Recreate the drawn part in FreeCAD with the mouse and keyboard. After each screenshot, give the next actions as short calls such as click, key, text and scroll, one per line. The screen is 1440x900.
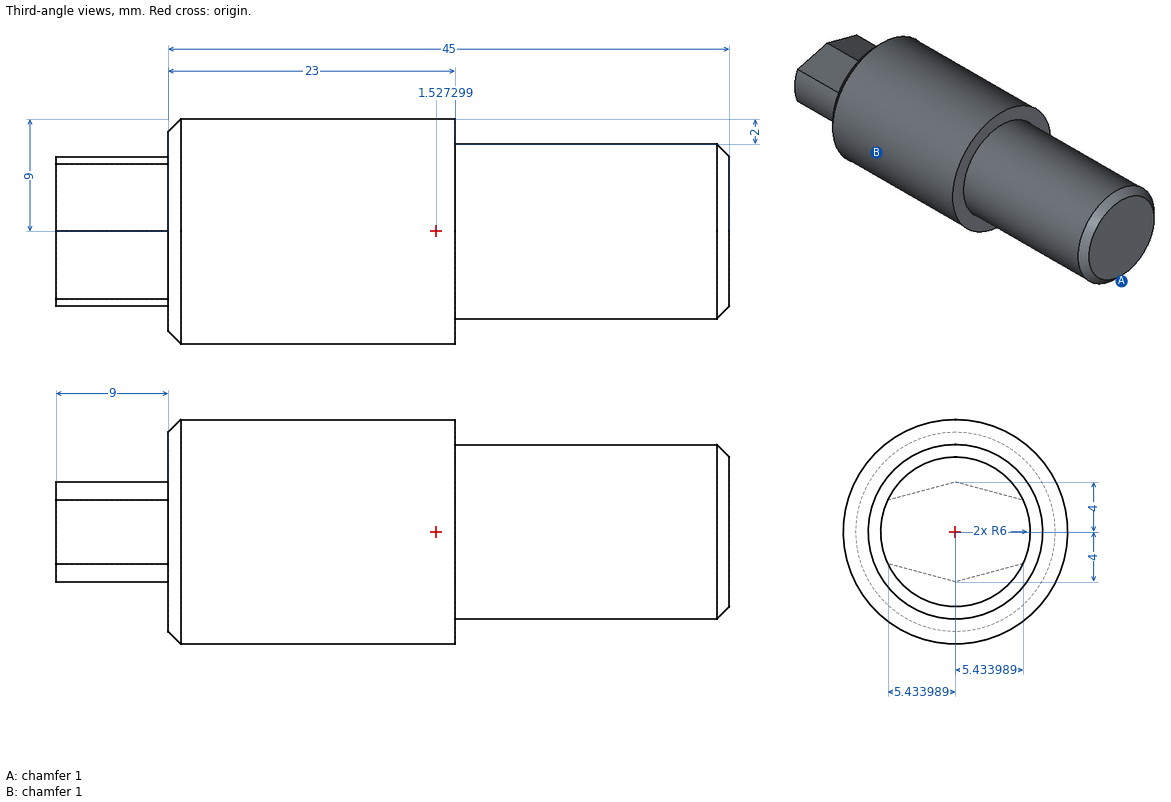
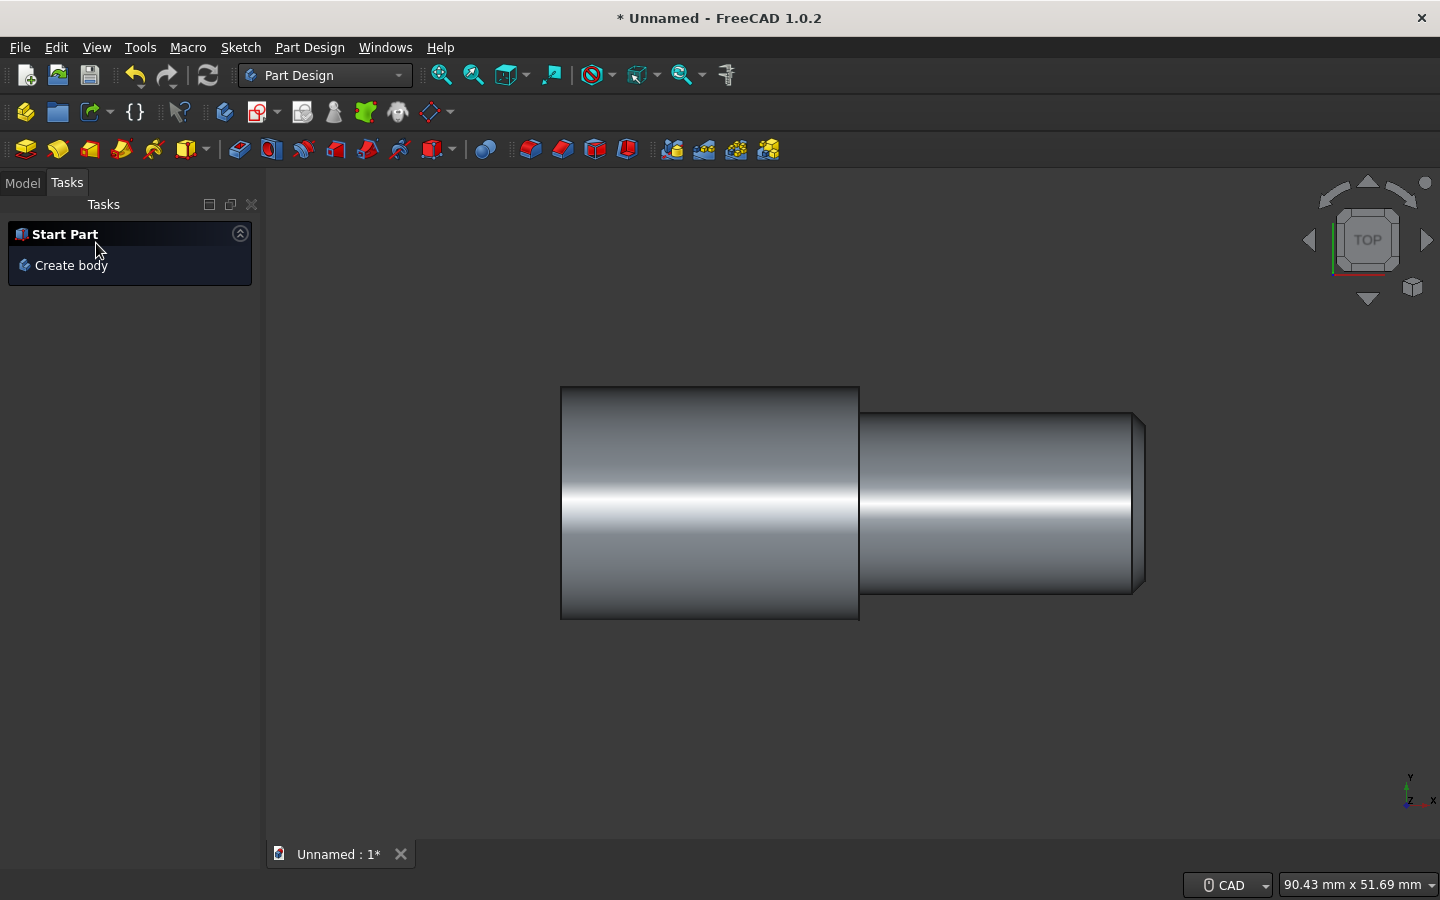
click(561, 597)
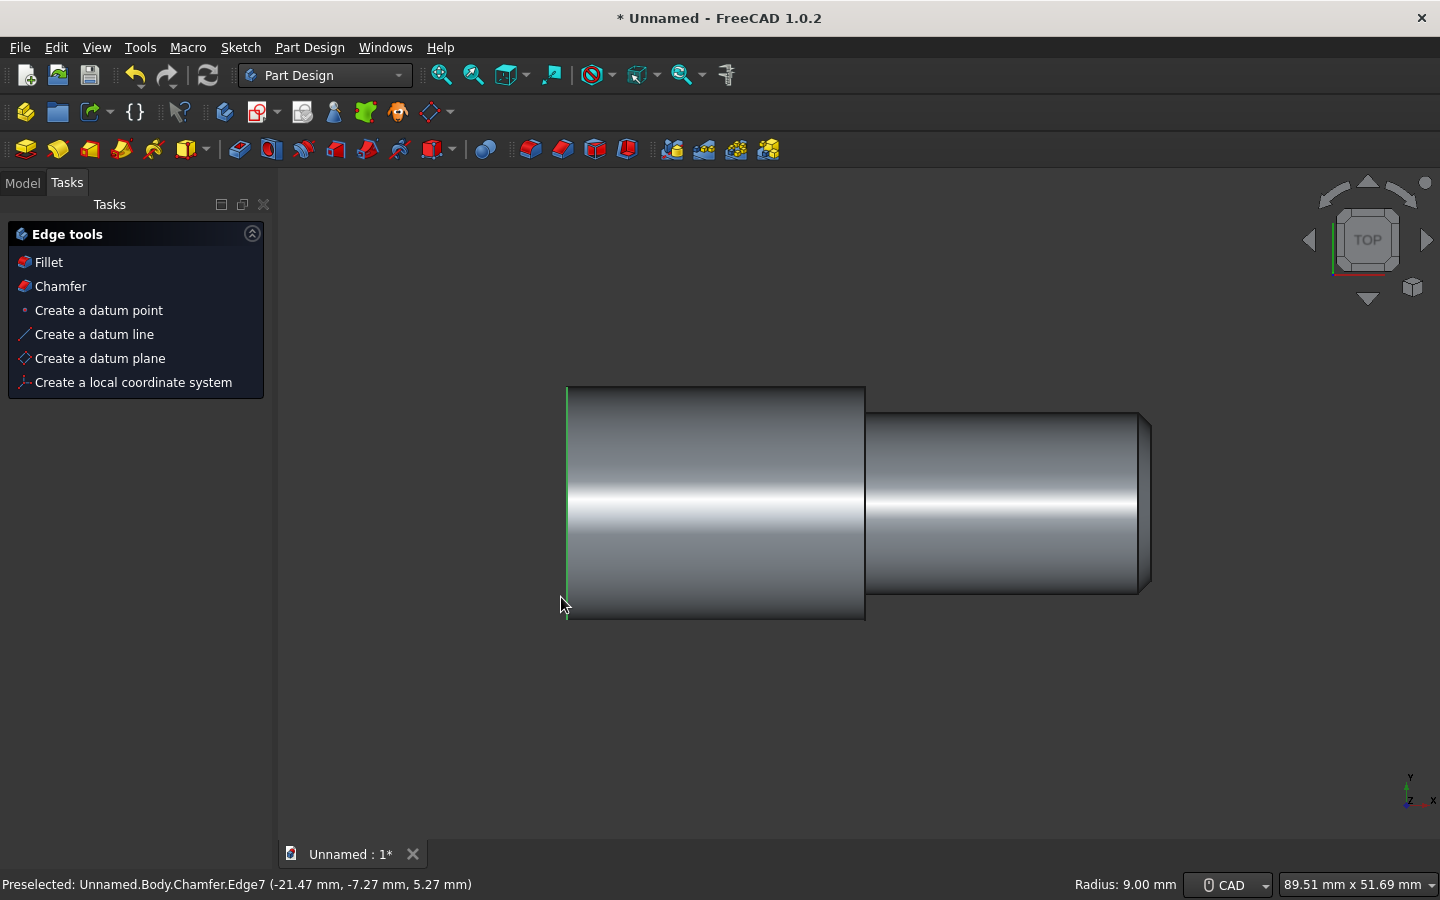
click(564, 150)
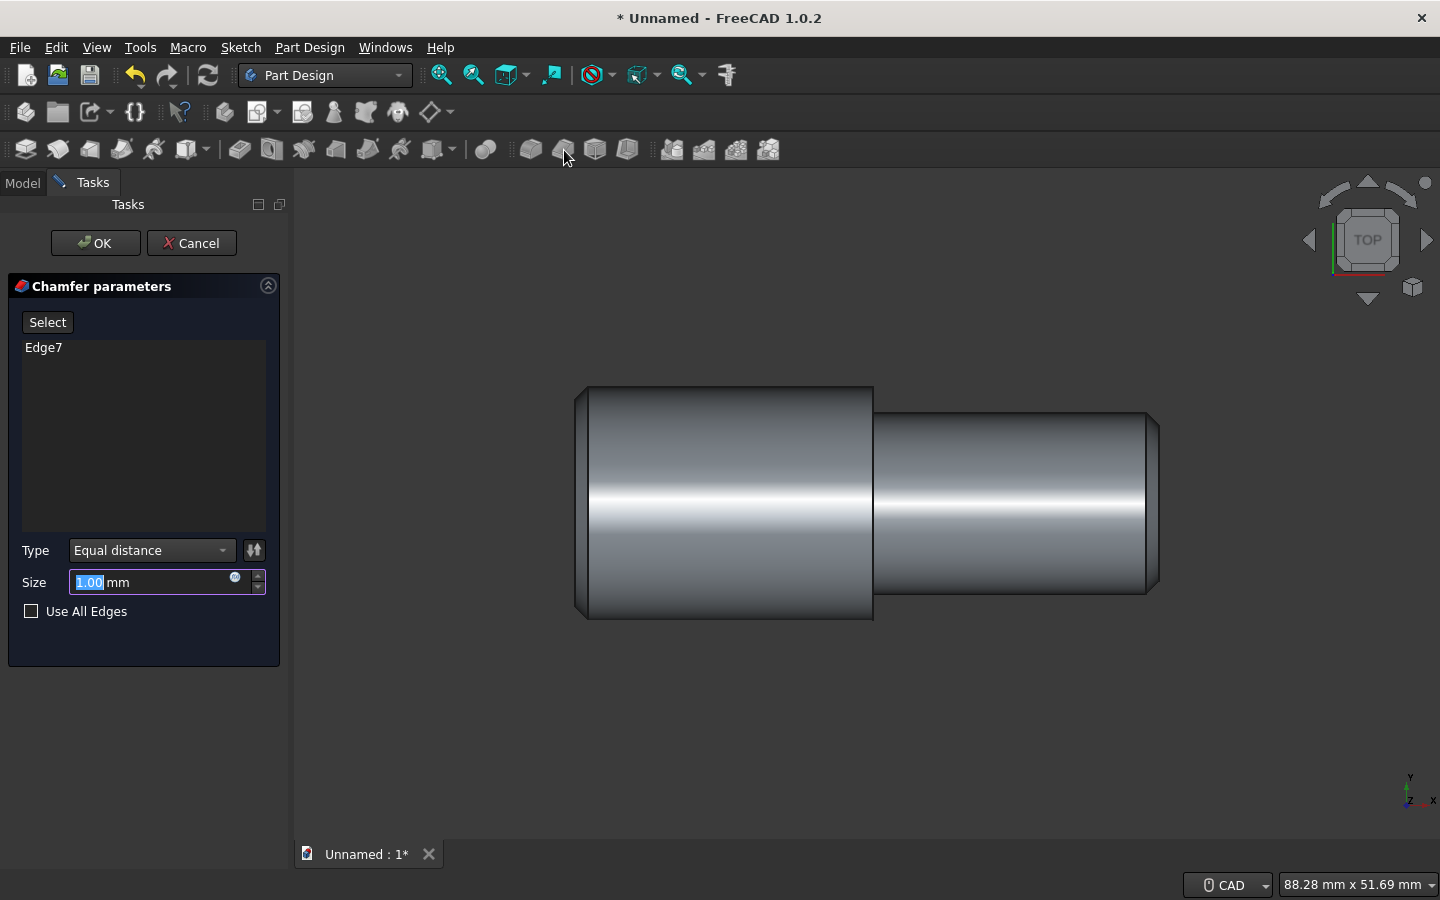
text(1)
key(Tab)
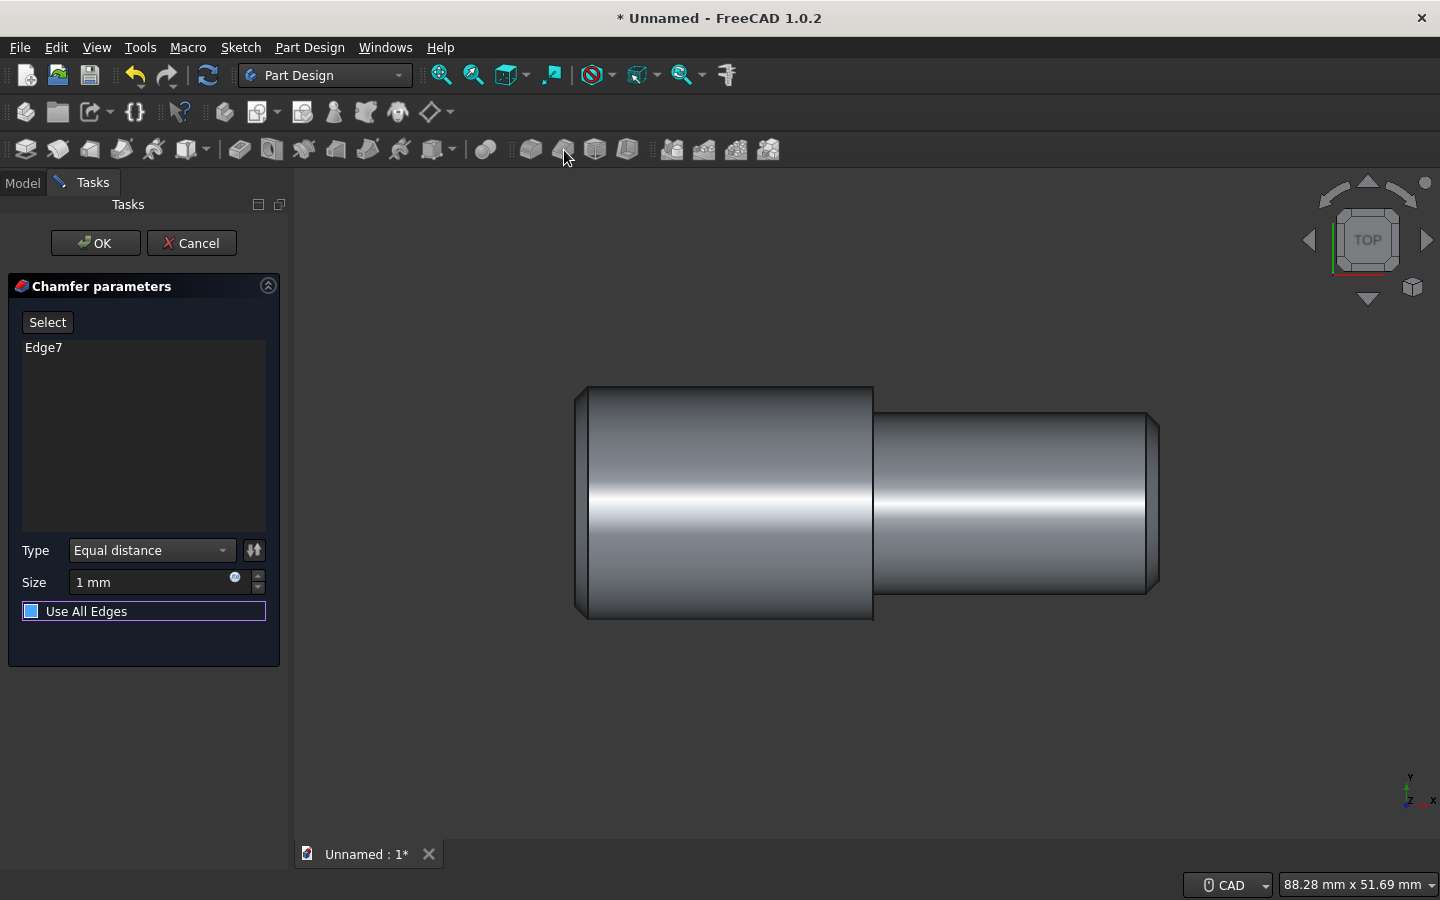
click(96, 243)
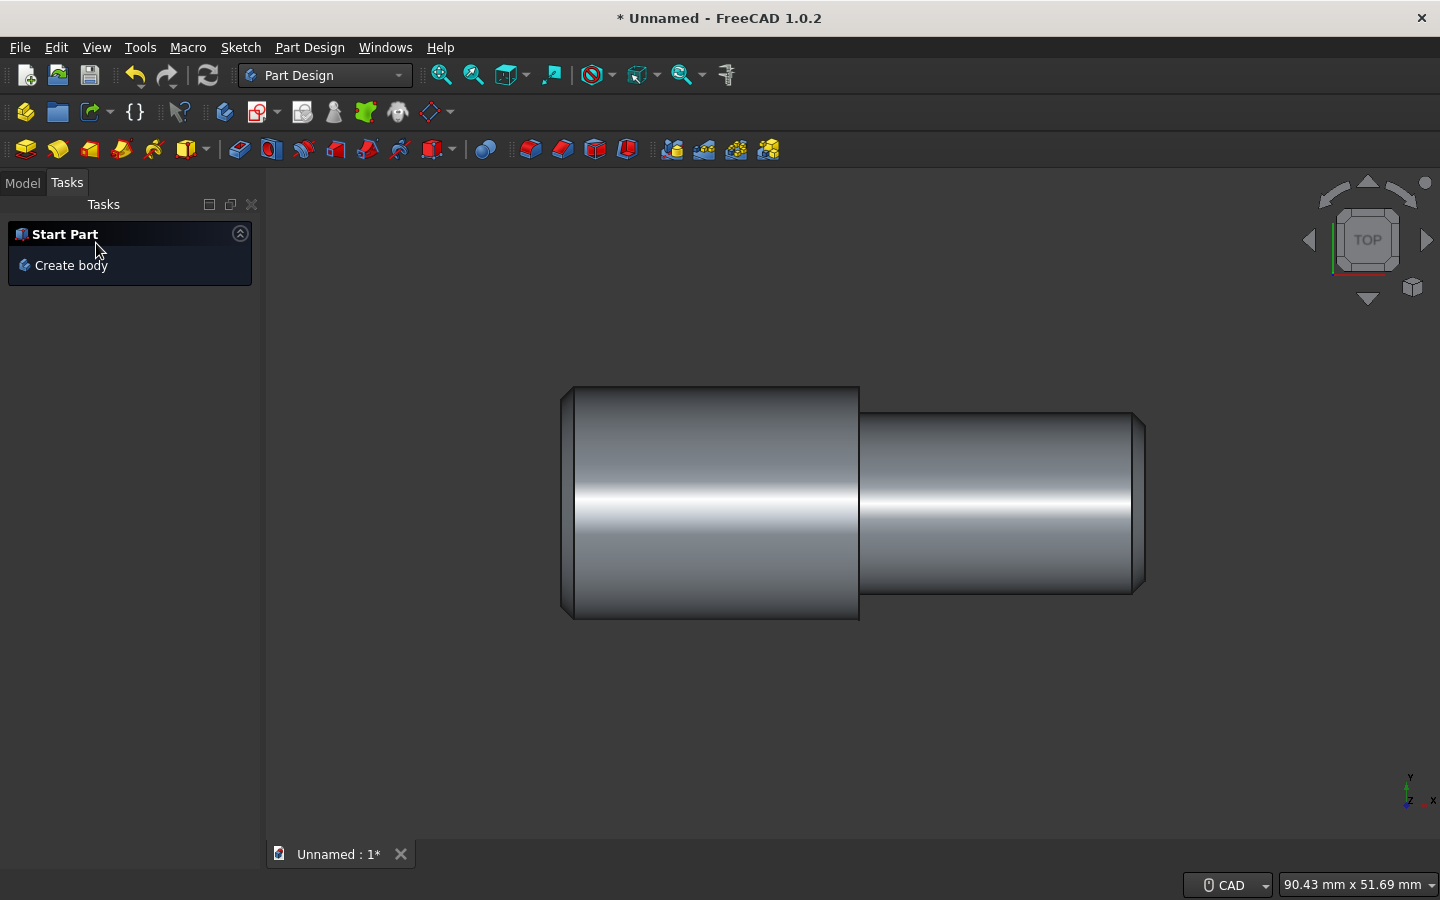
key(6)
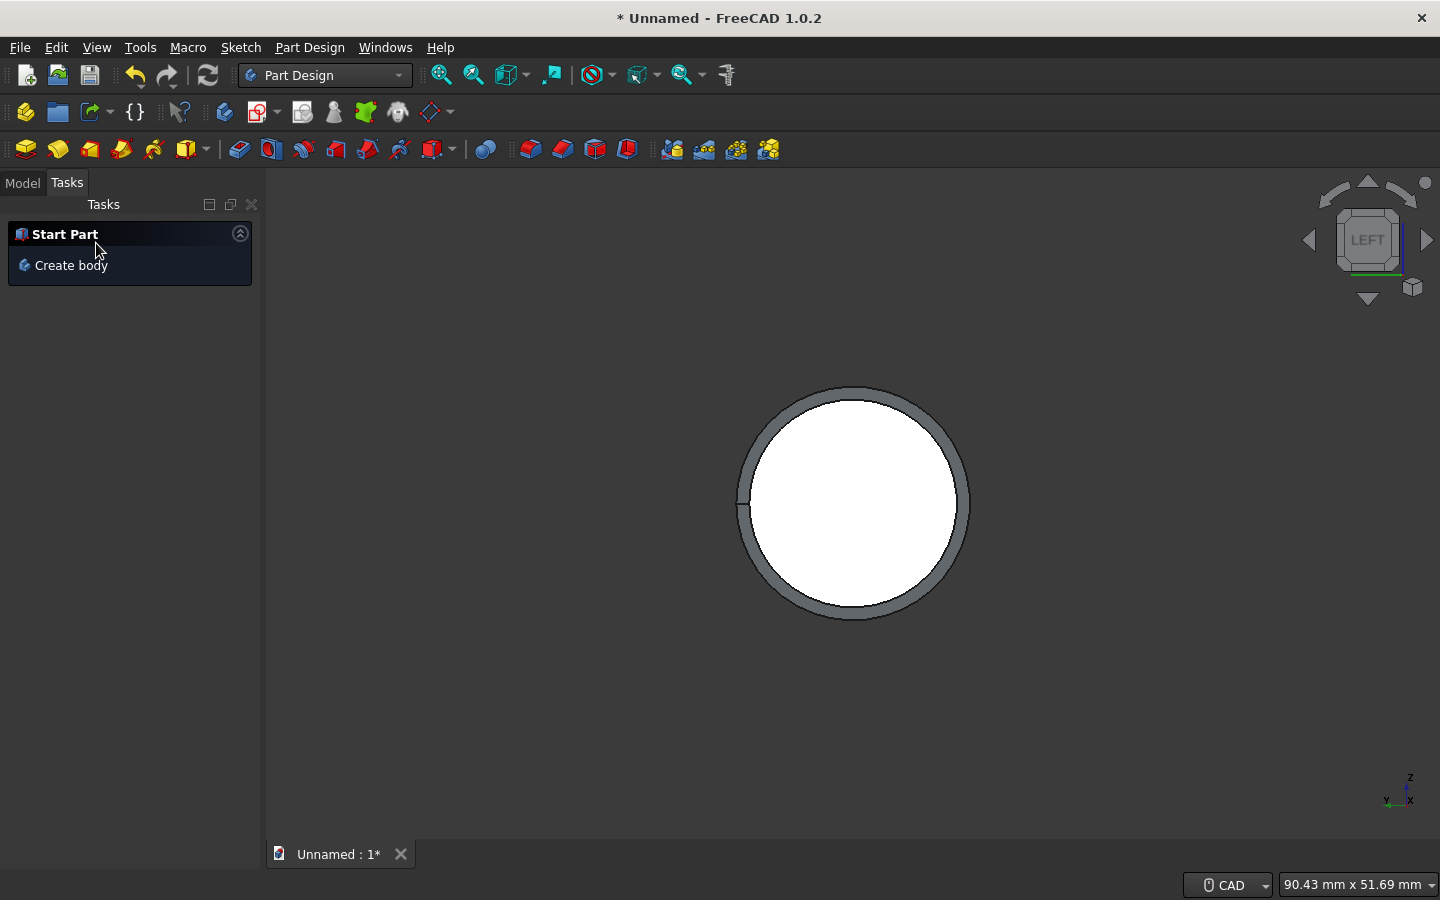
click(442, 76)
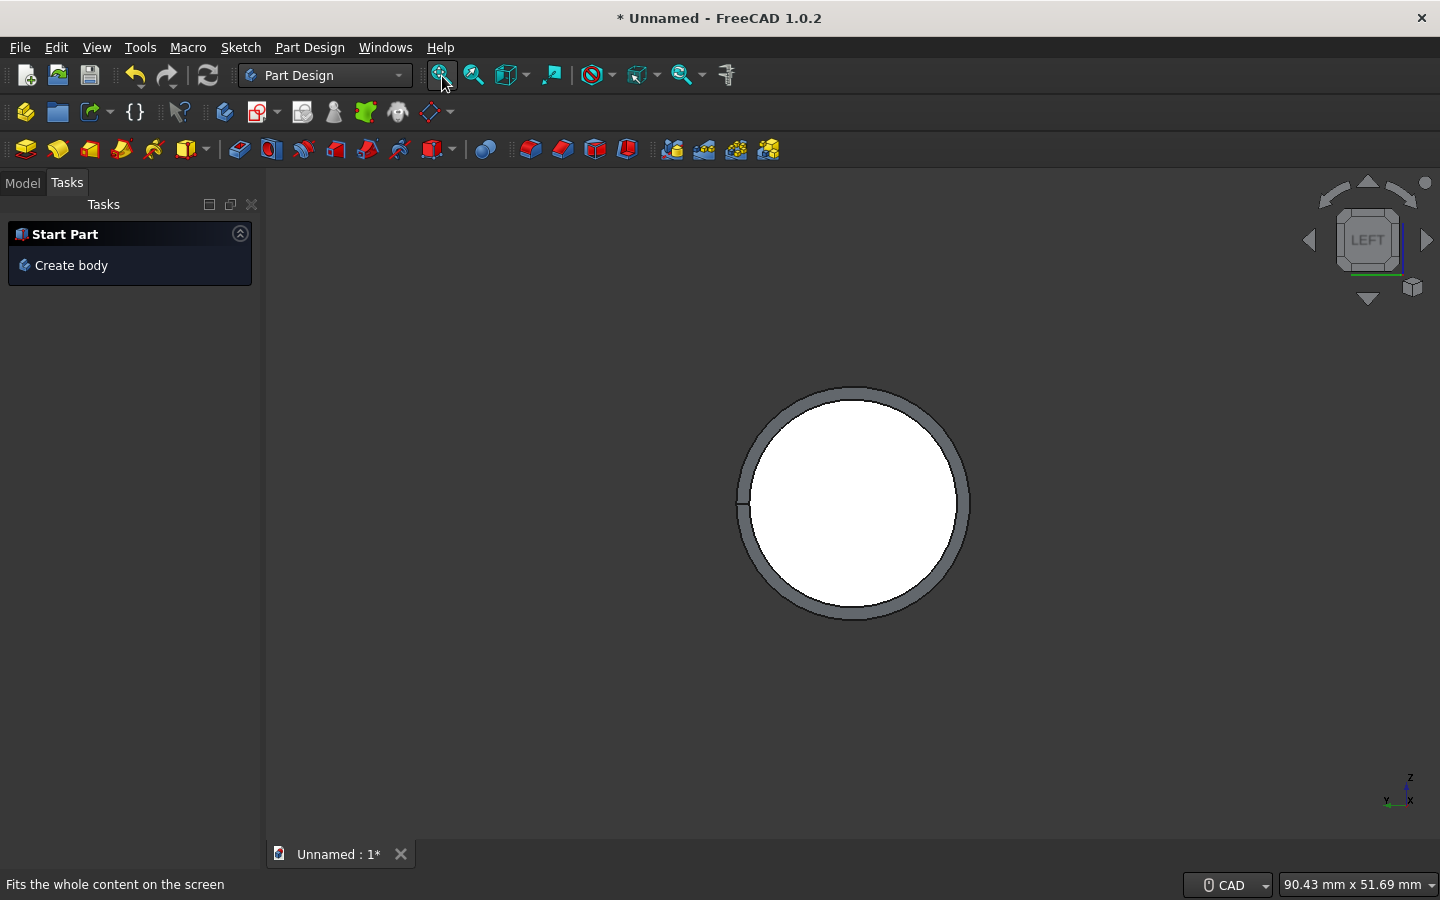
click(853, 502)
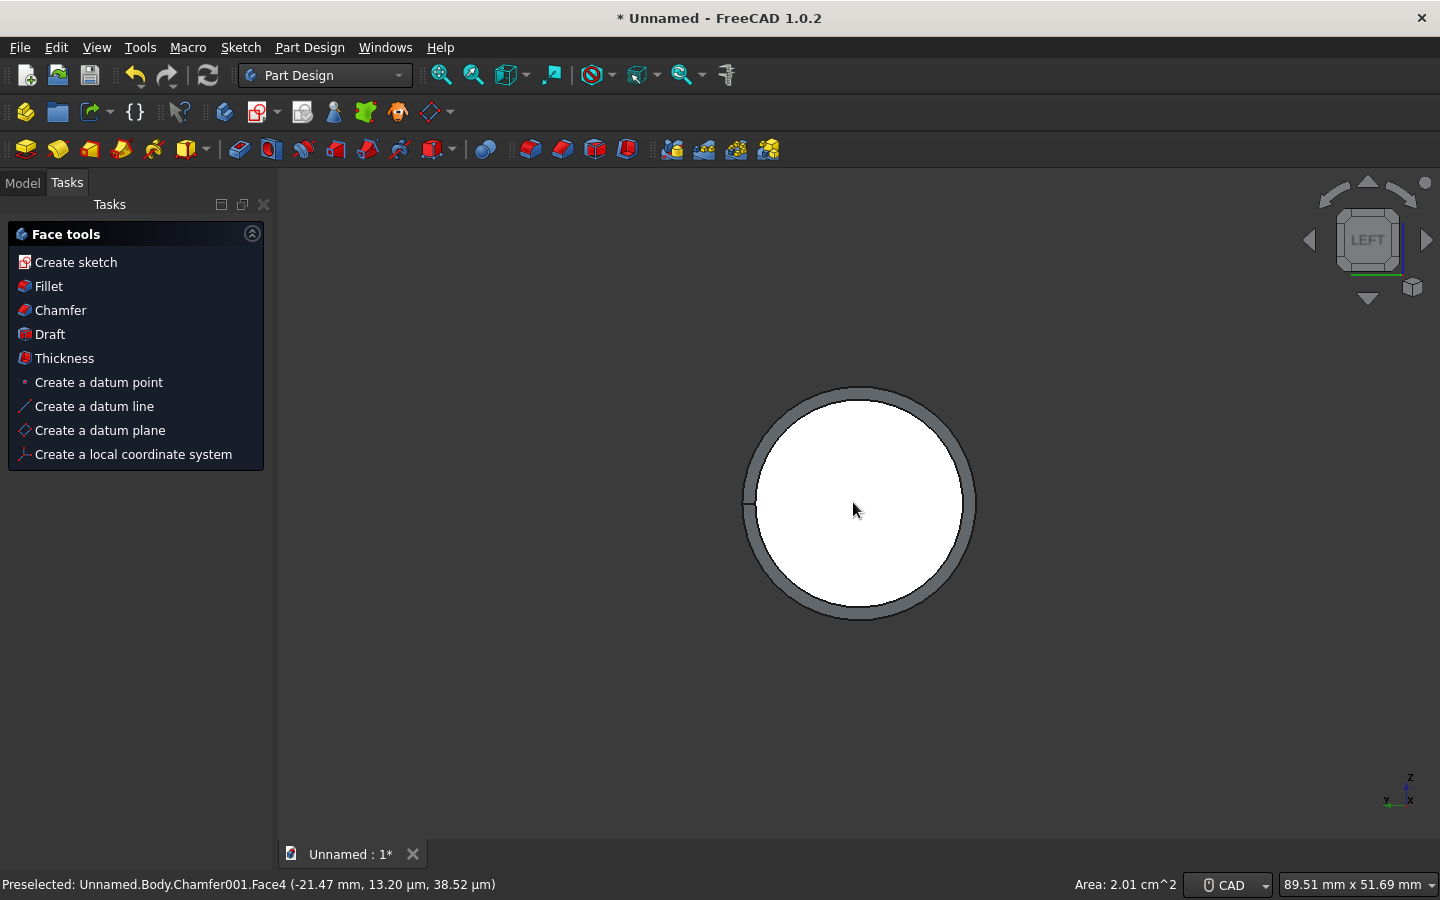
click(258, 112)